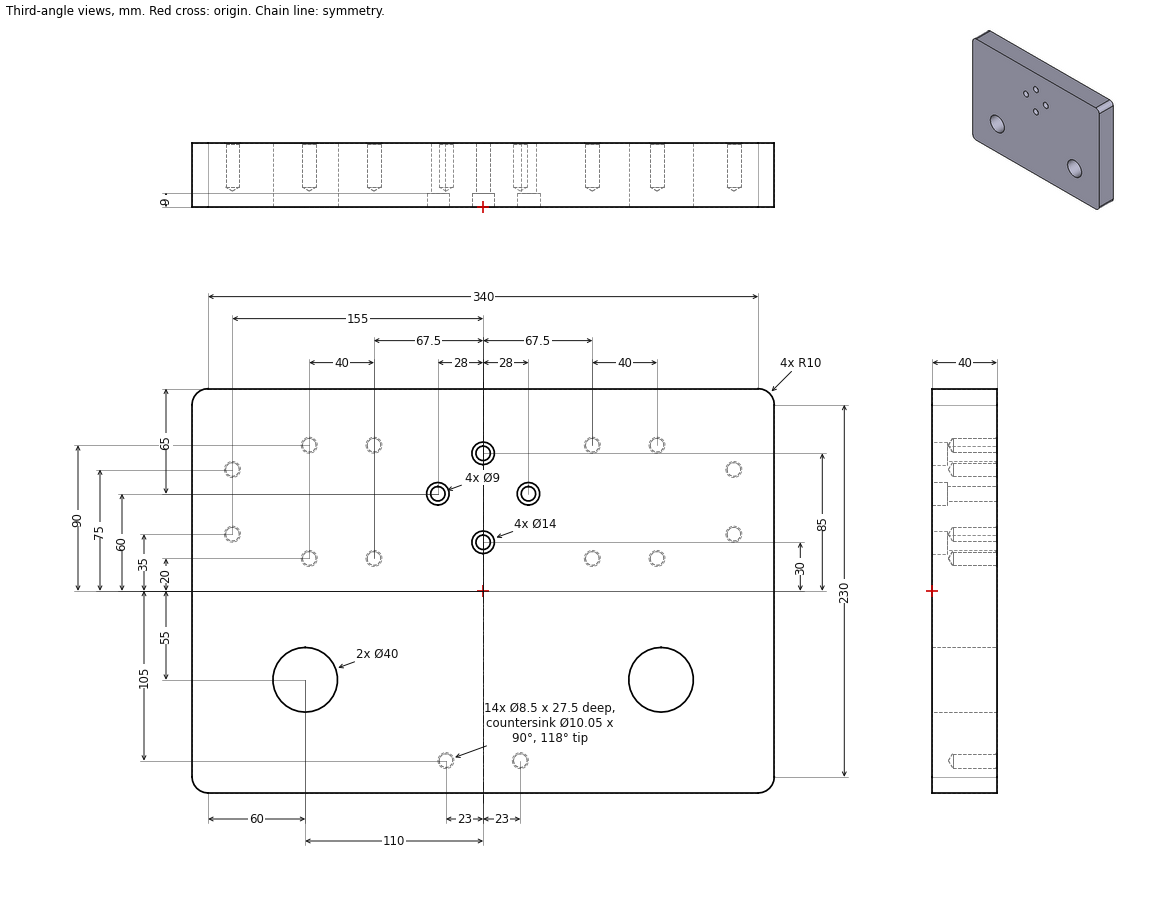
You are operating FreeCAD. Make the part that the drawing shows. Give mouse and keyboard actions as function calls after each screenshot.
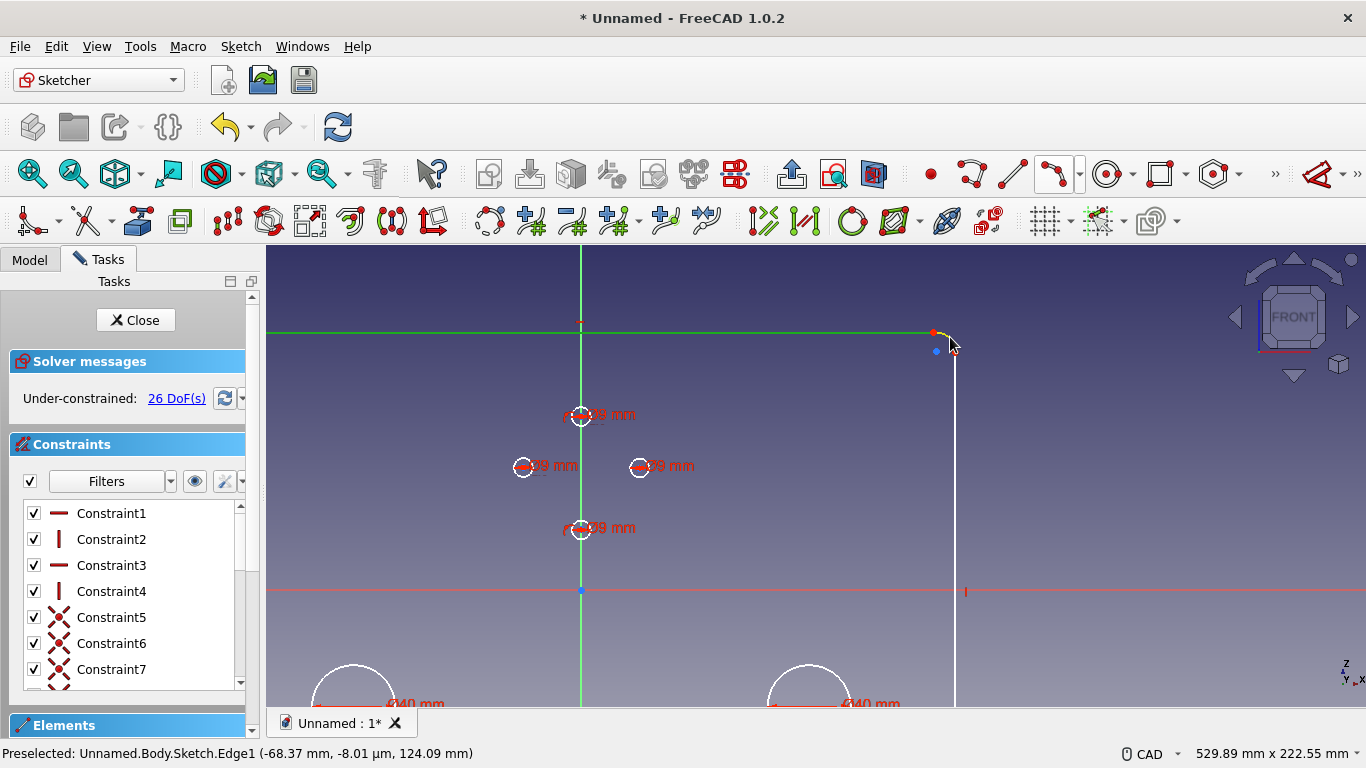
click(949, 338)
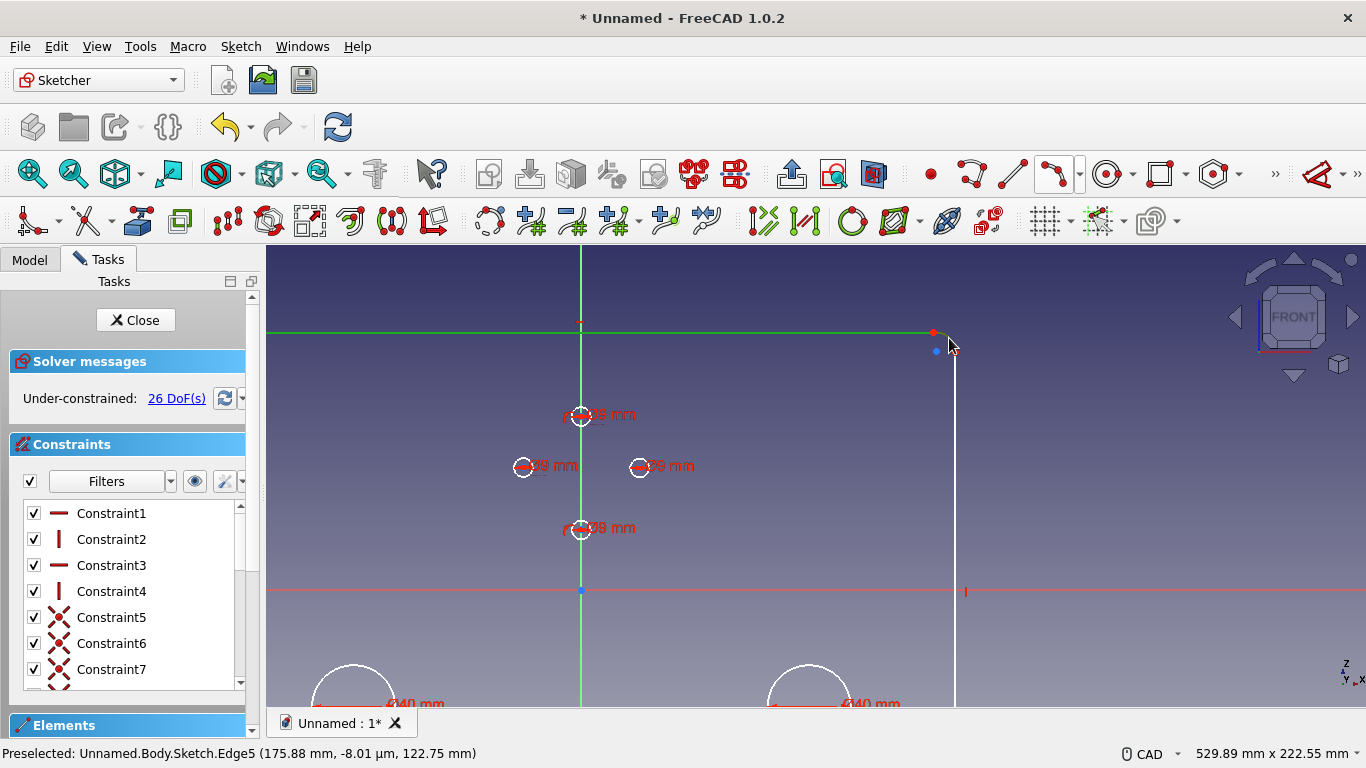
key(t)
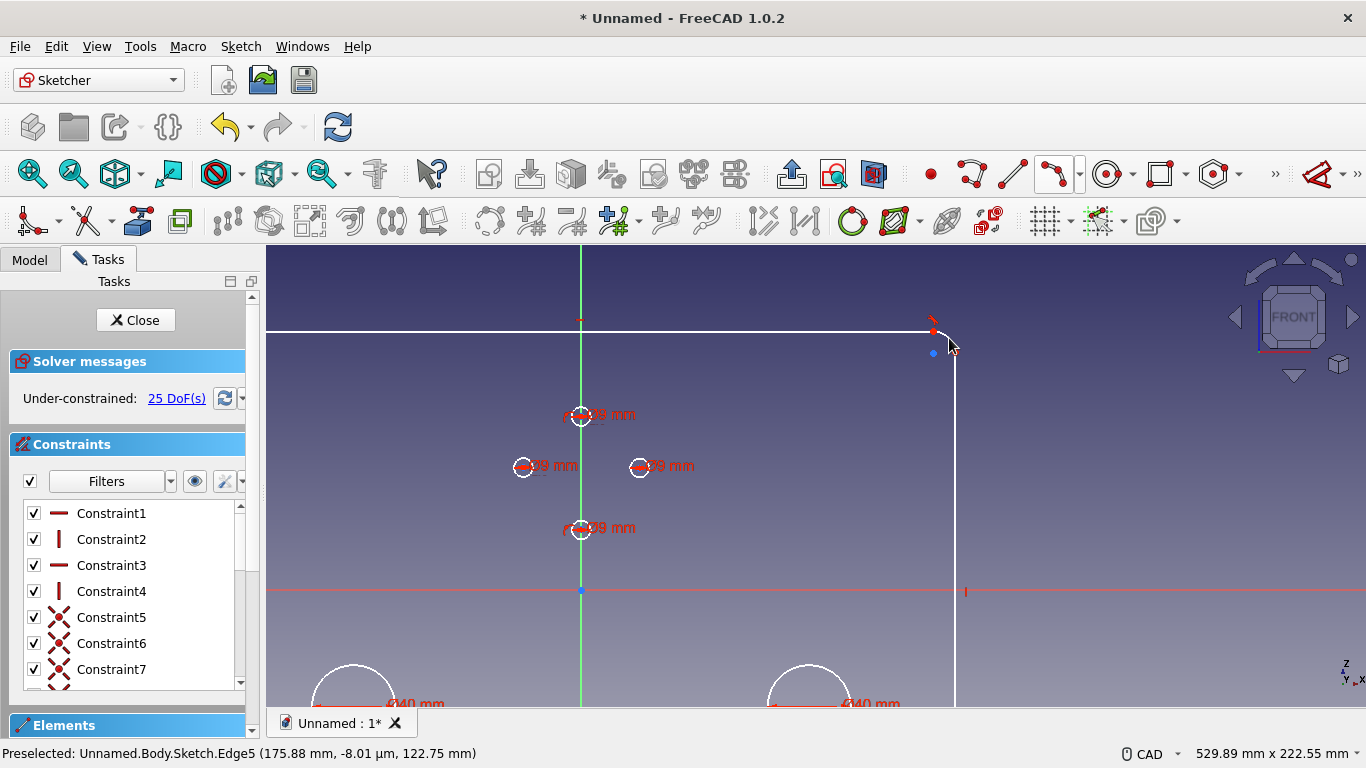
click(440, 332)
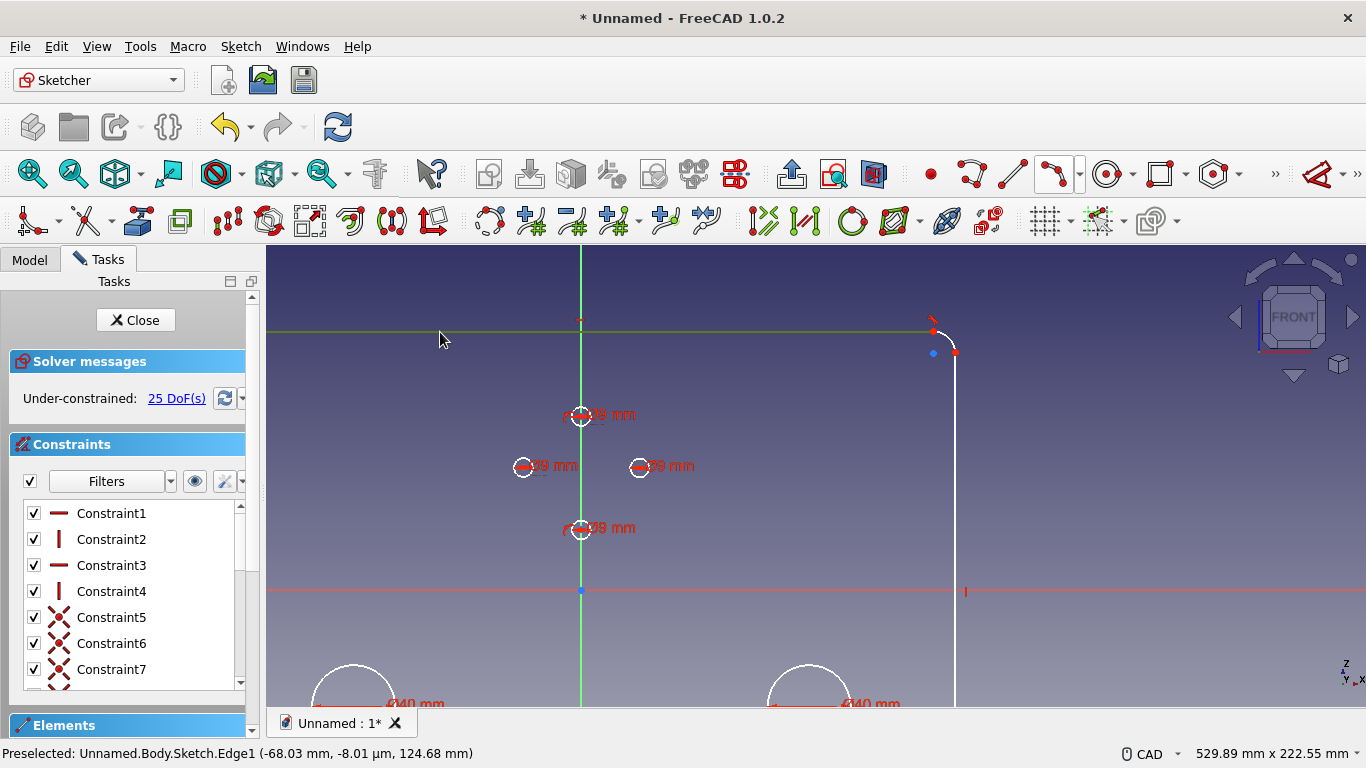
scroll(950, 337, down, 3)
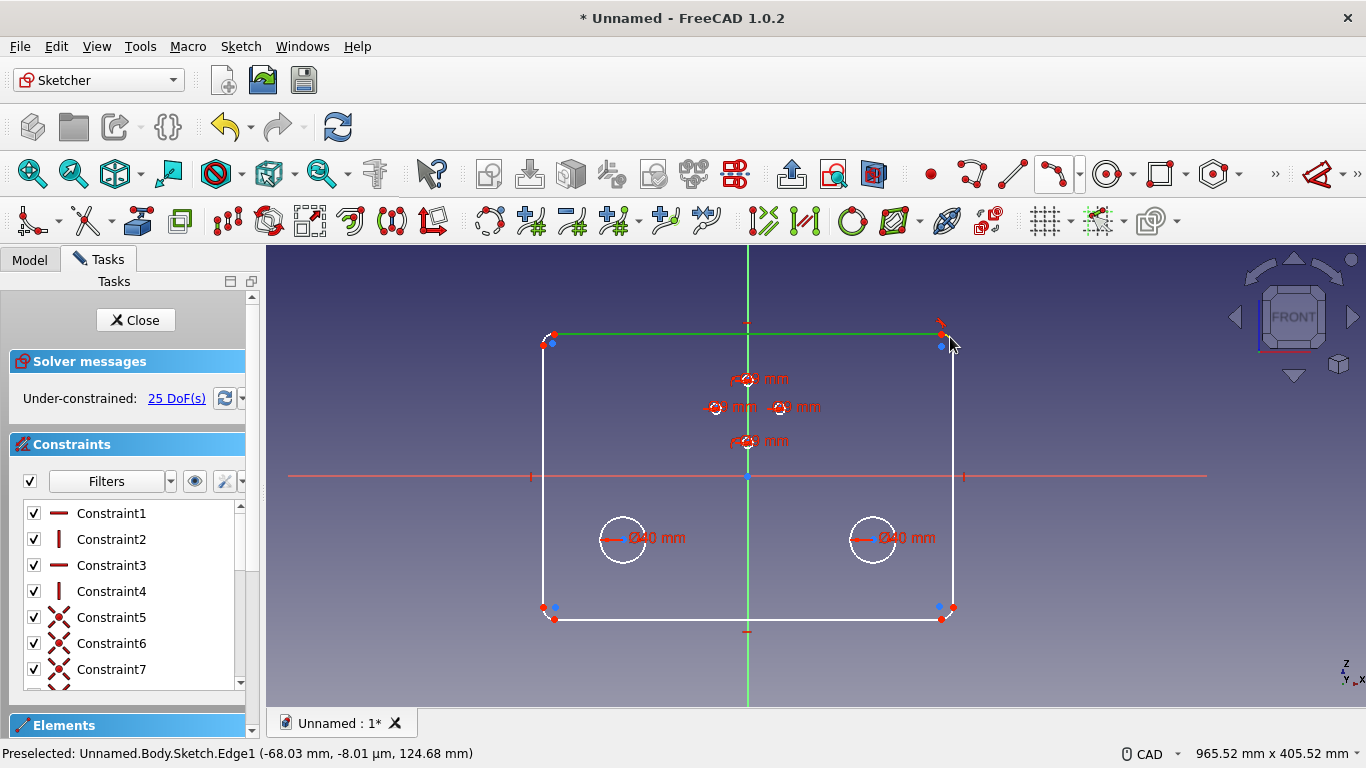
scroll(549, 335, up, 5)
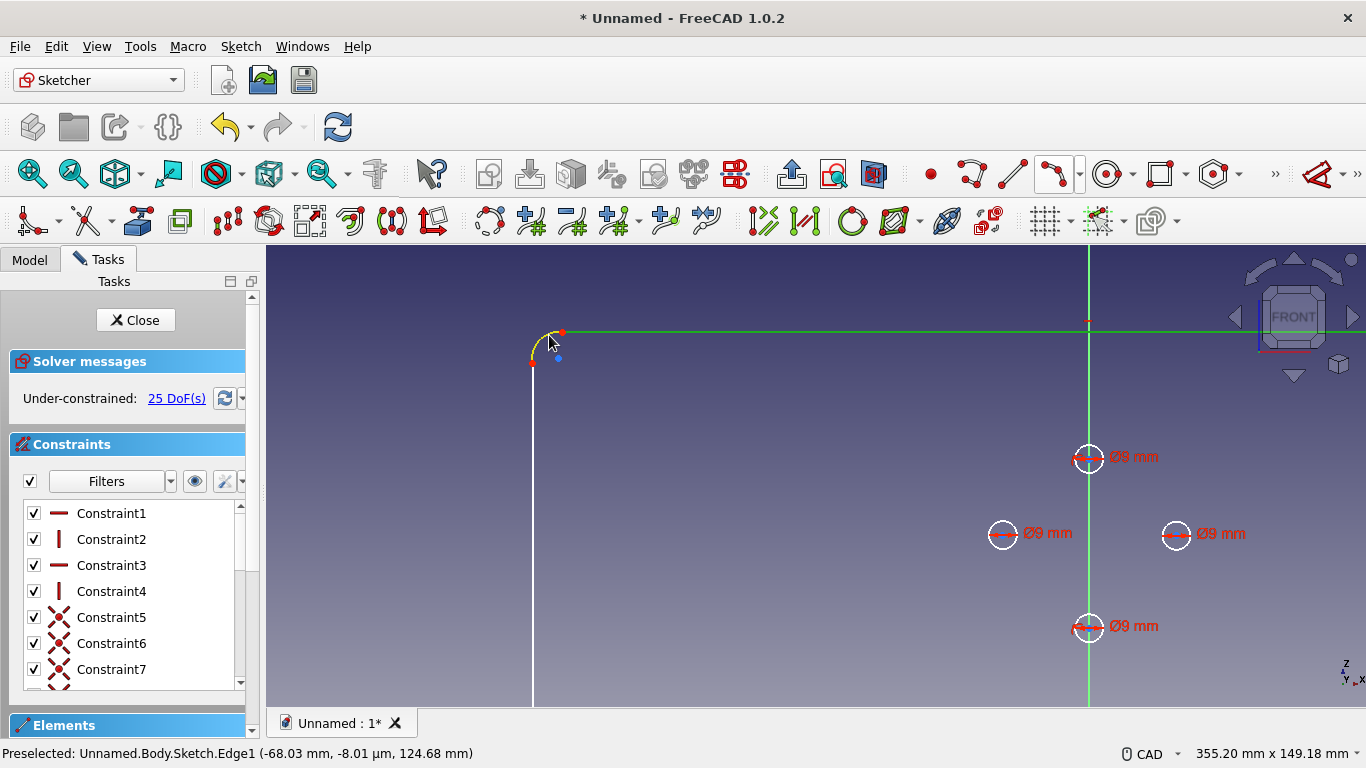
click(548, 334)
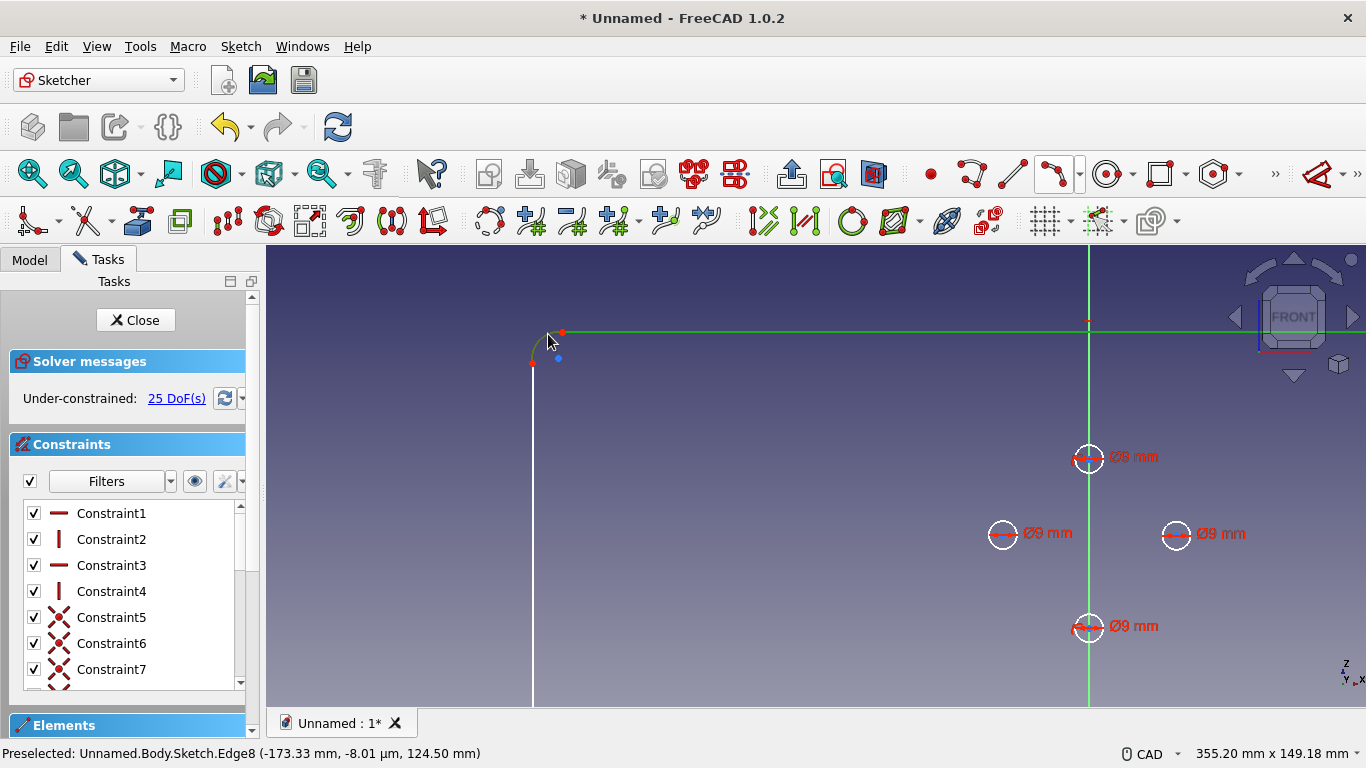
key(t)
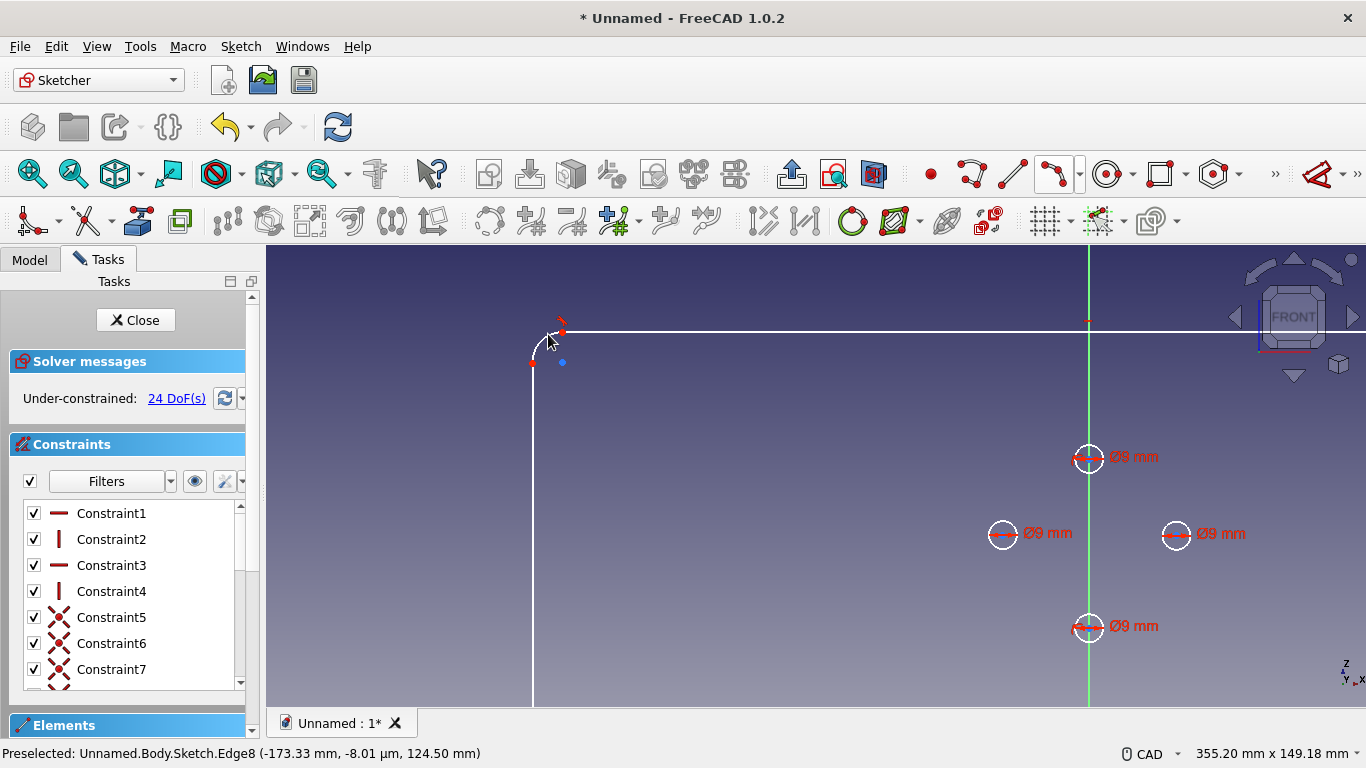
scroll(549, 335, down, 5)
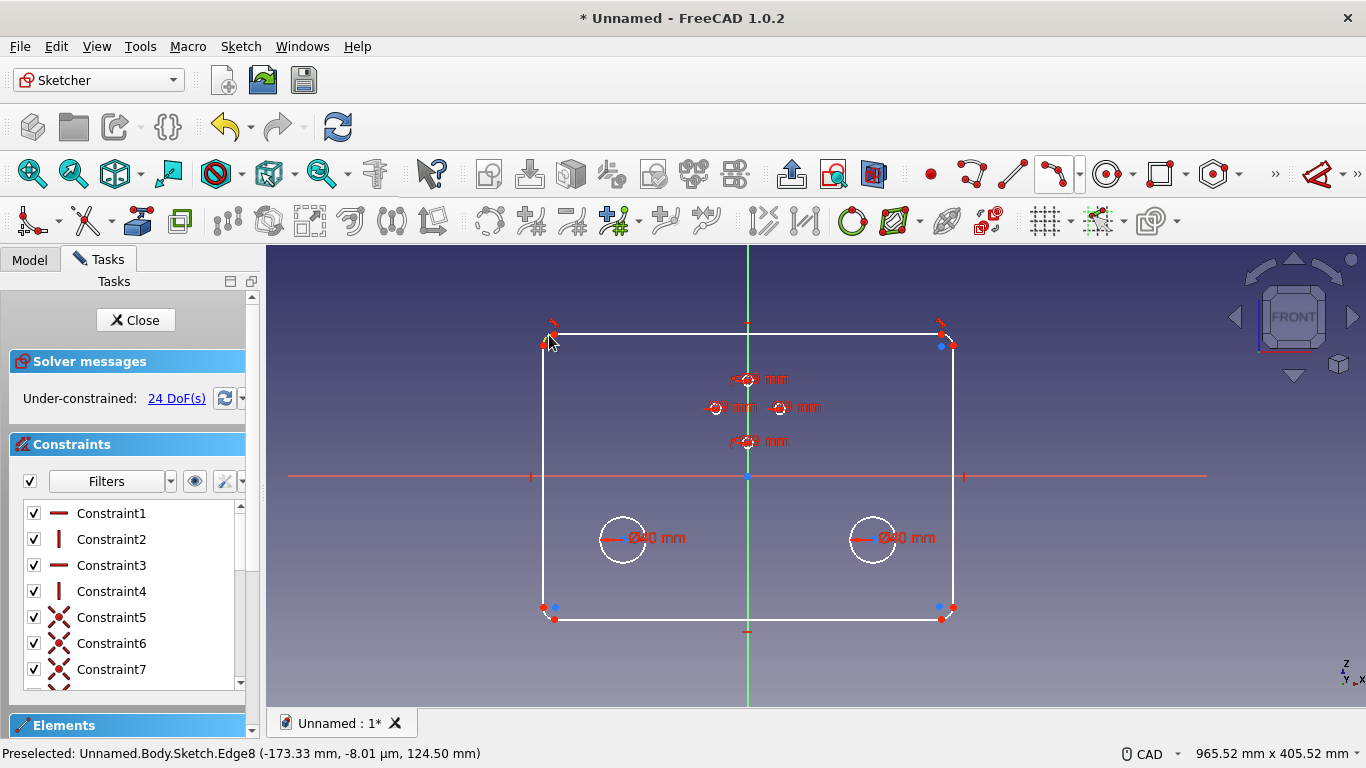
click(953, 424)